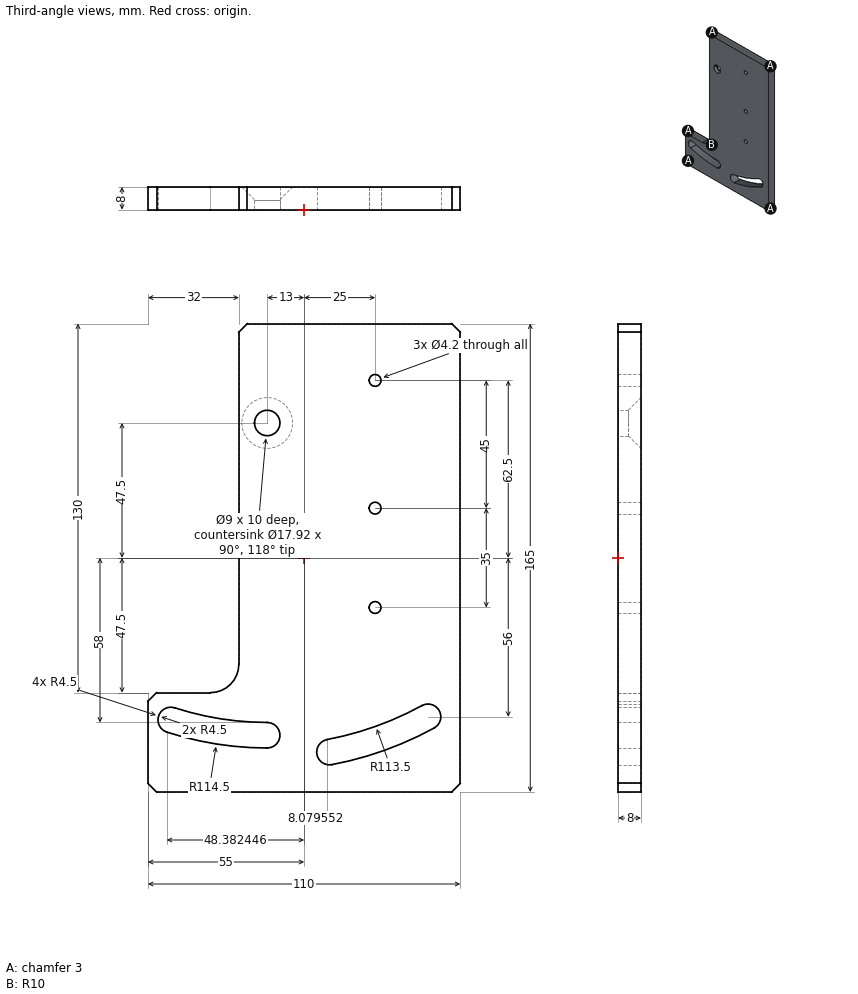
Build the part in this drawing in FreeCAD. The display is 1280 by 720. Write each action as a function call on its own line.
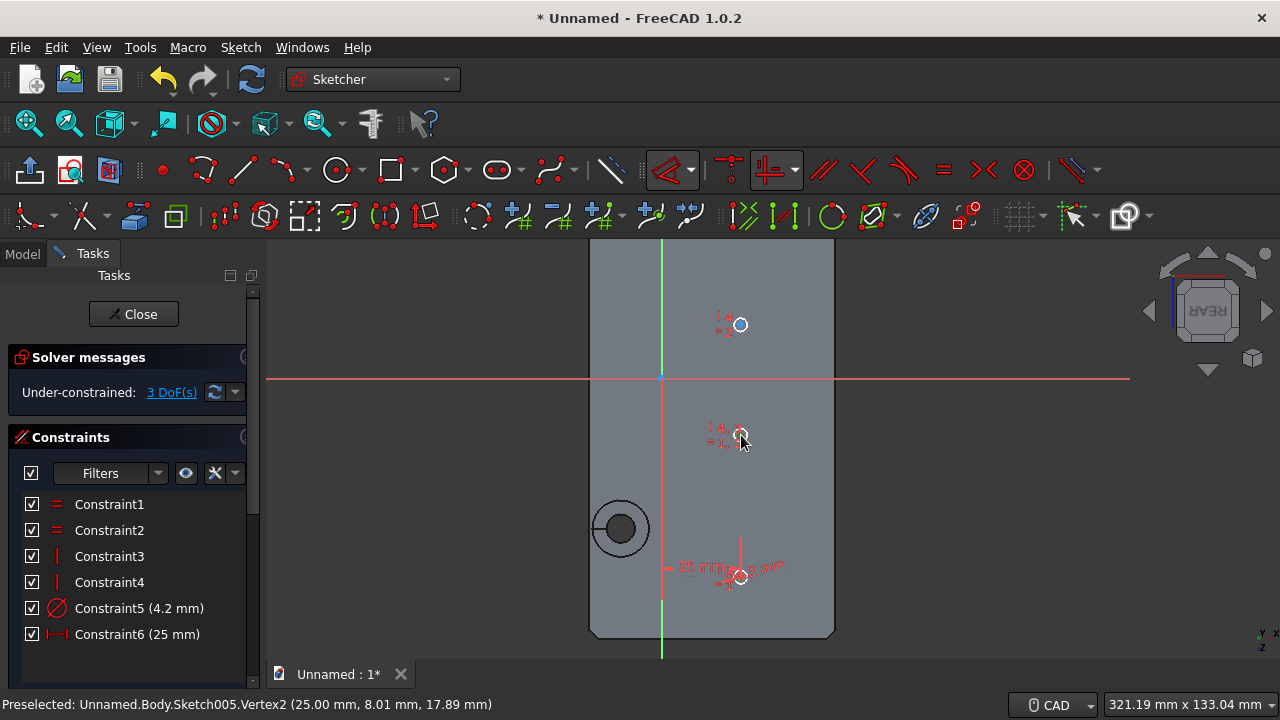
click(694, 170)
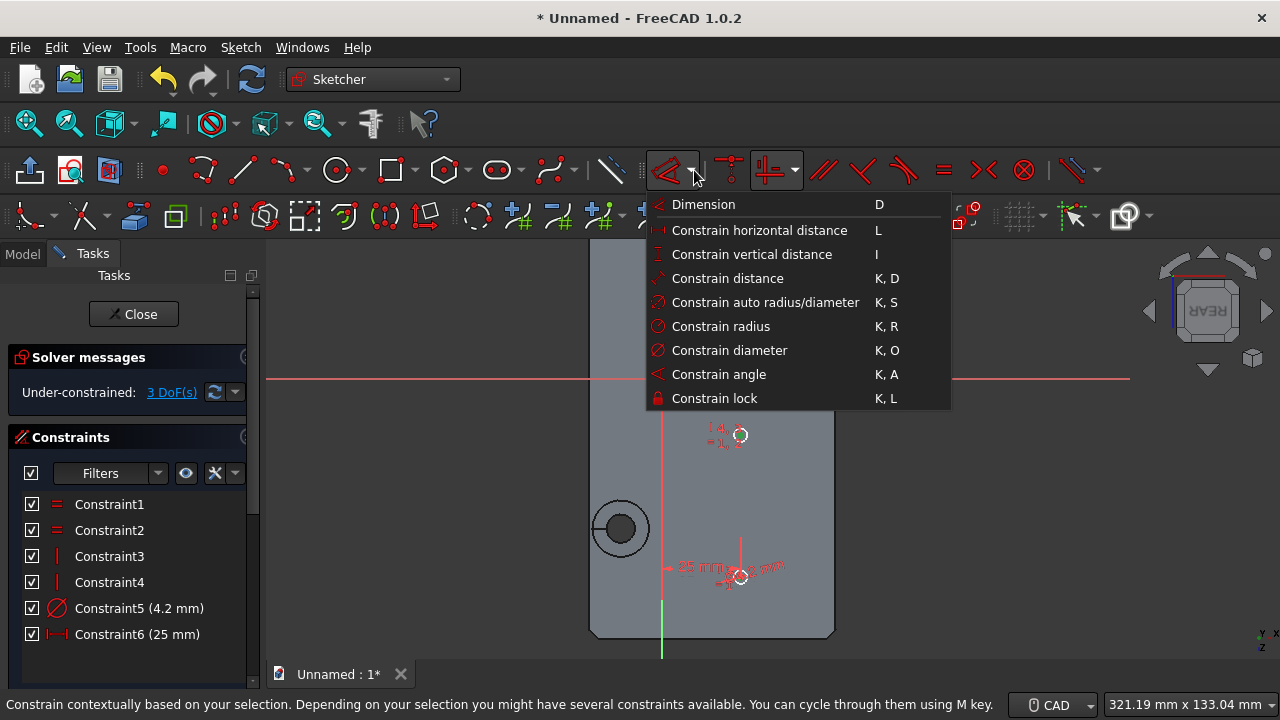
click(799, 254)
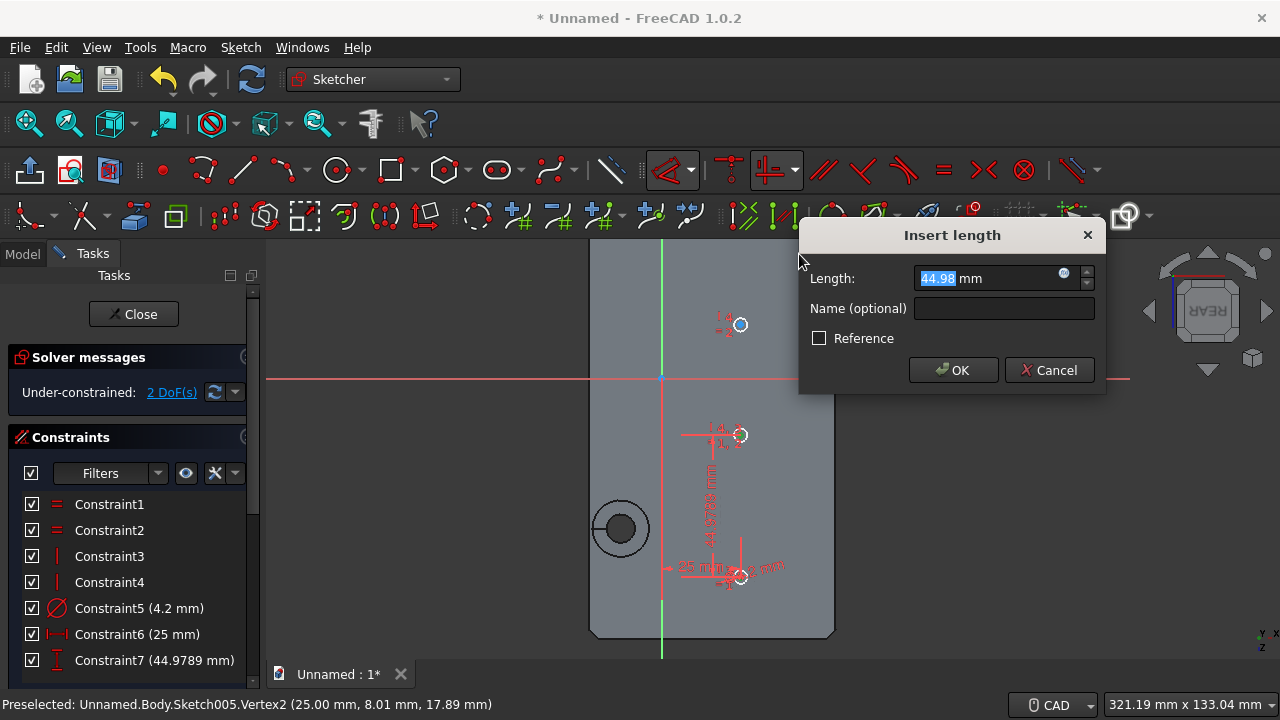
text(45)
key(Return)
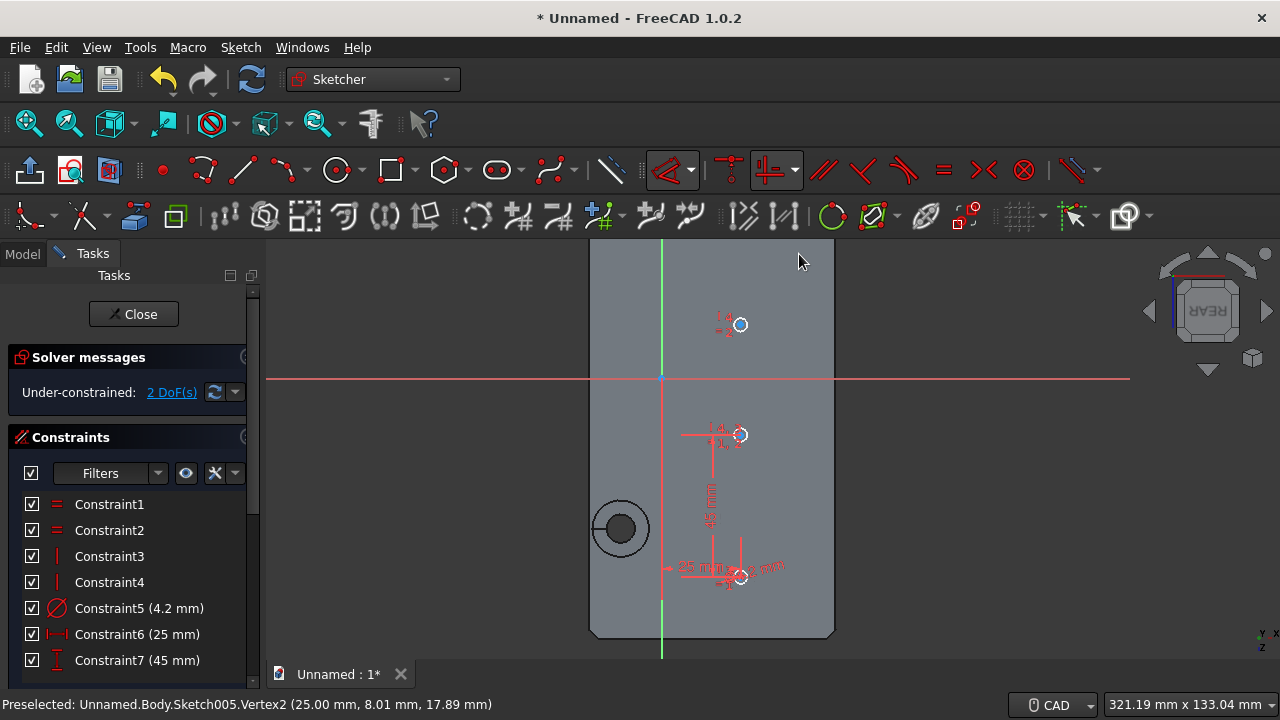
click(741, 435)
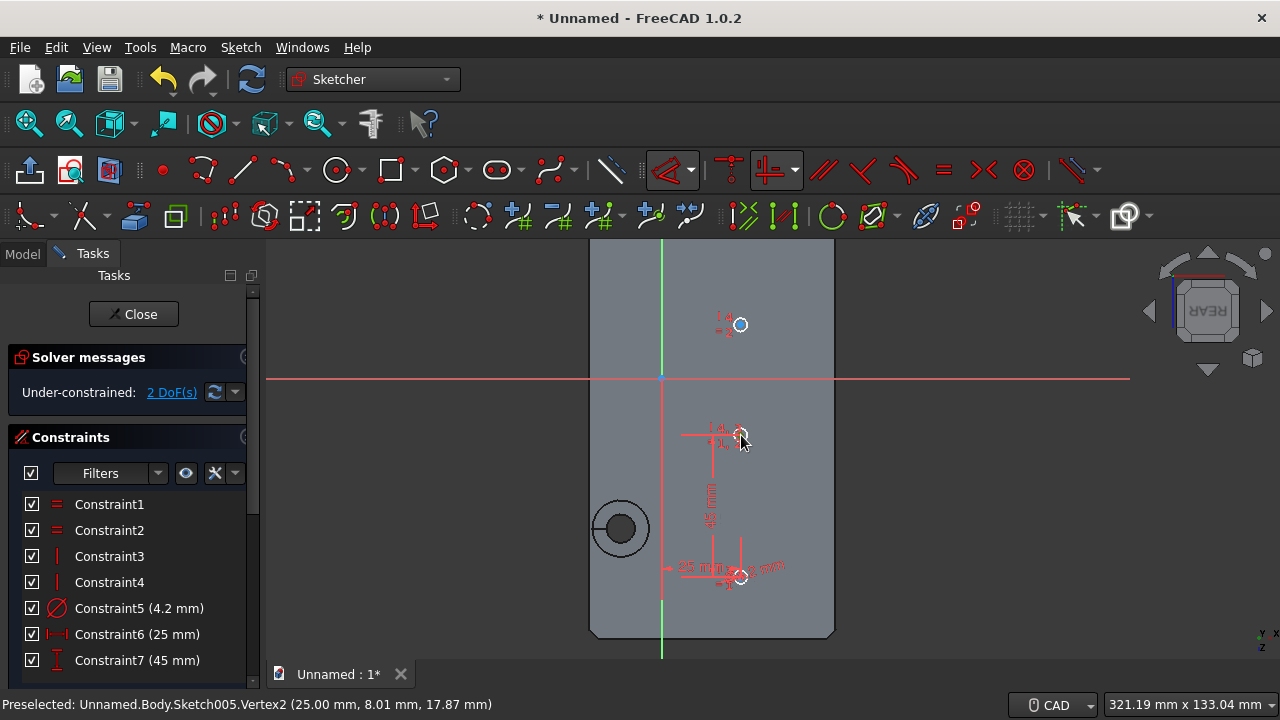
click(741, 325)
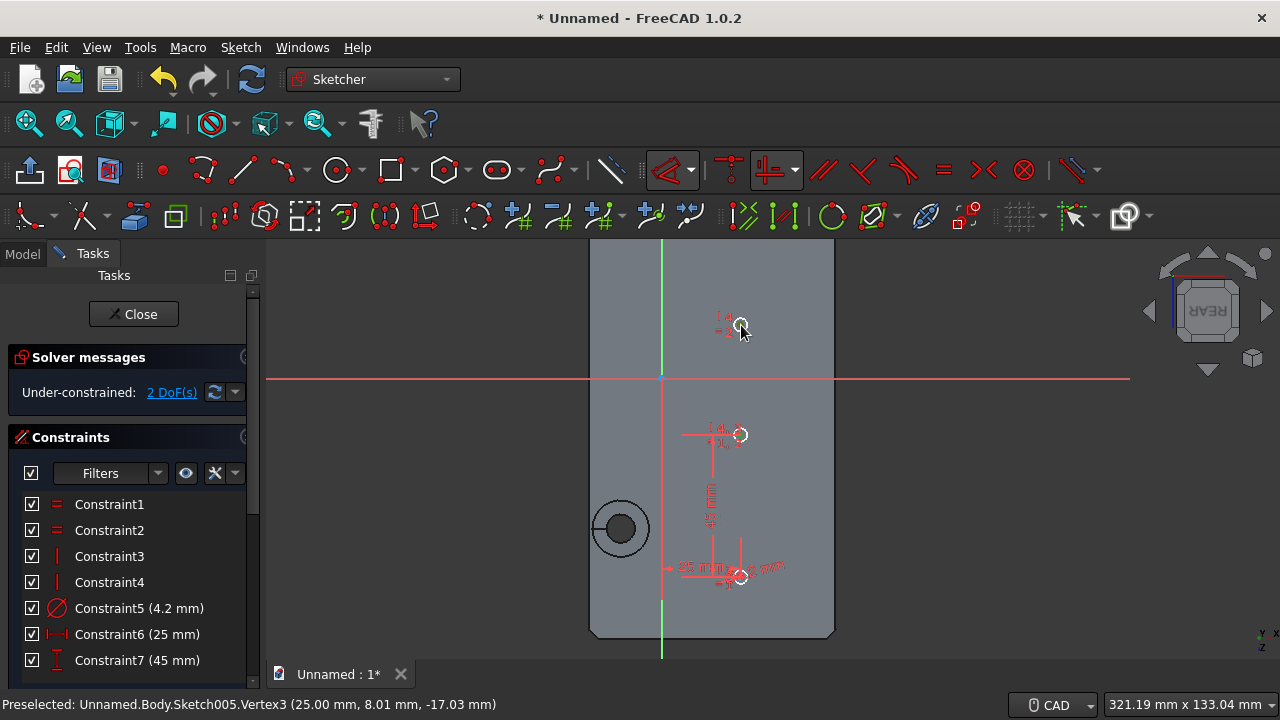
click(694, 170)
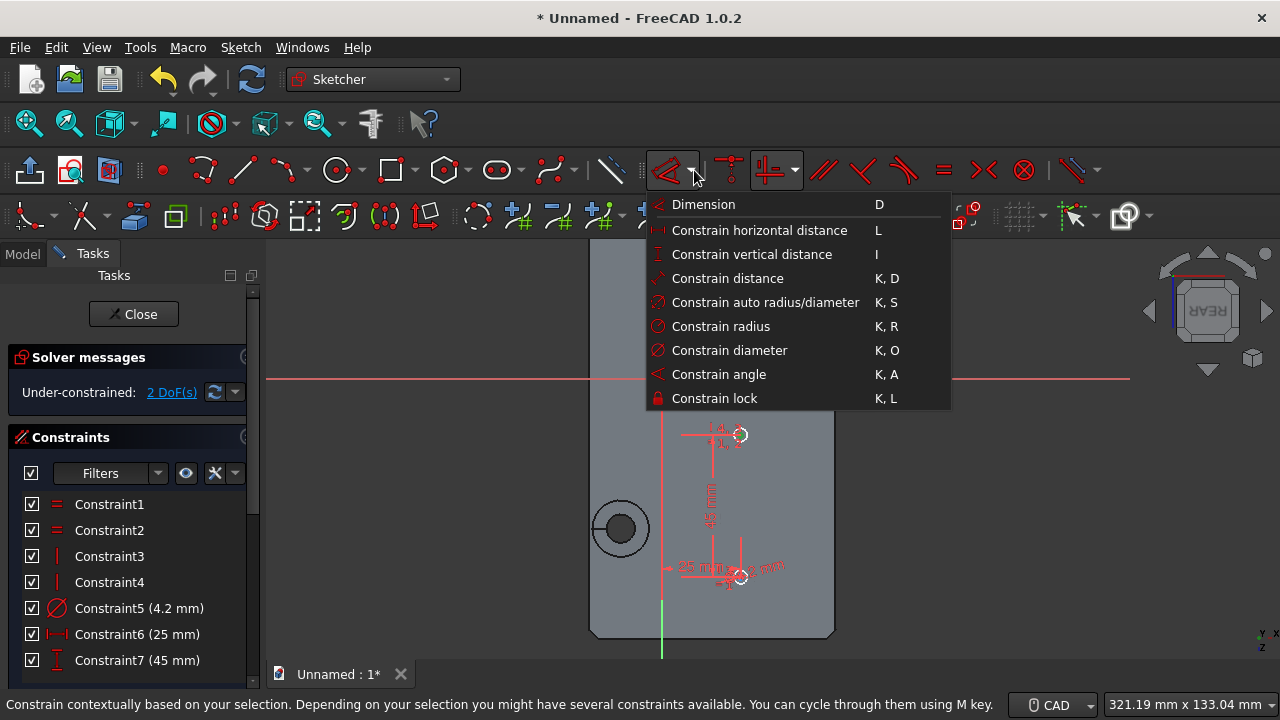
click(799, 254)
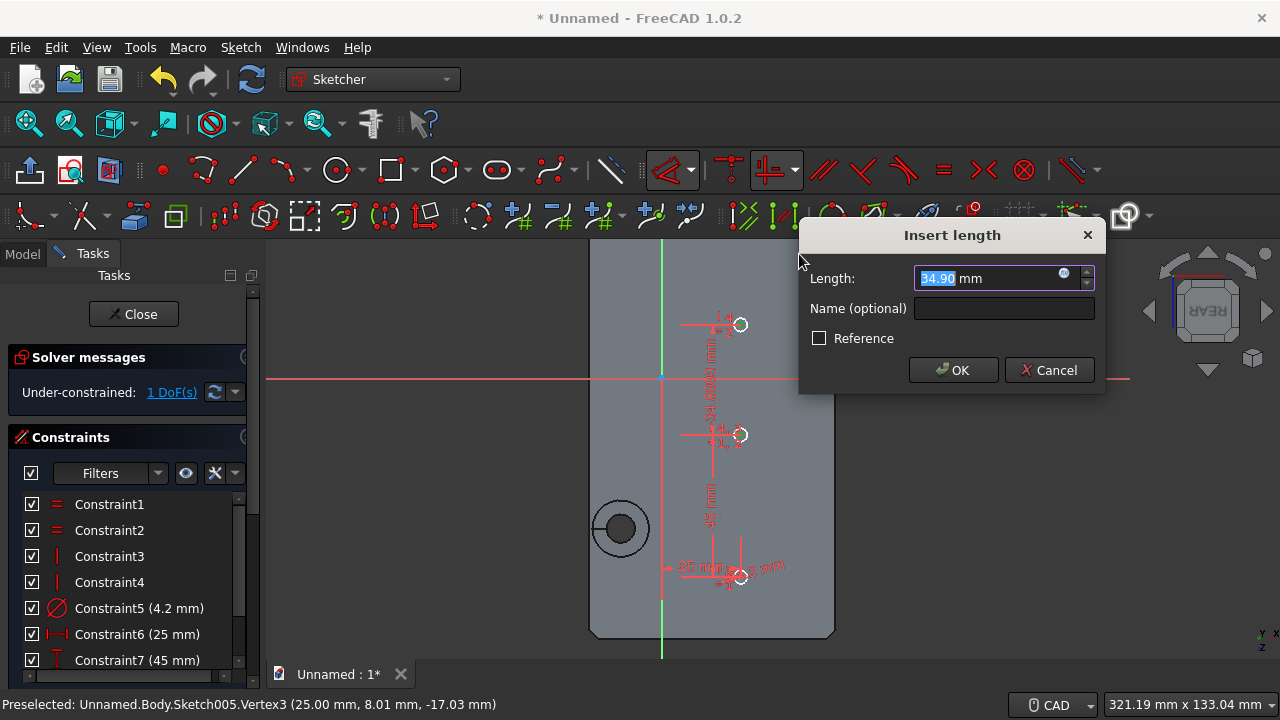
text(35)
key(Return)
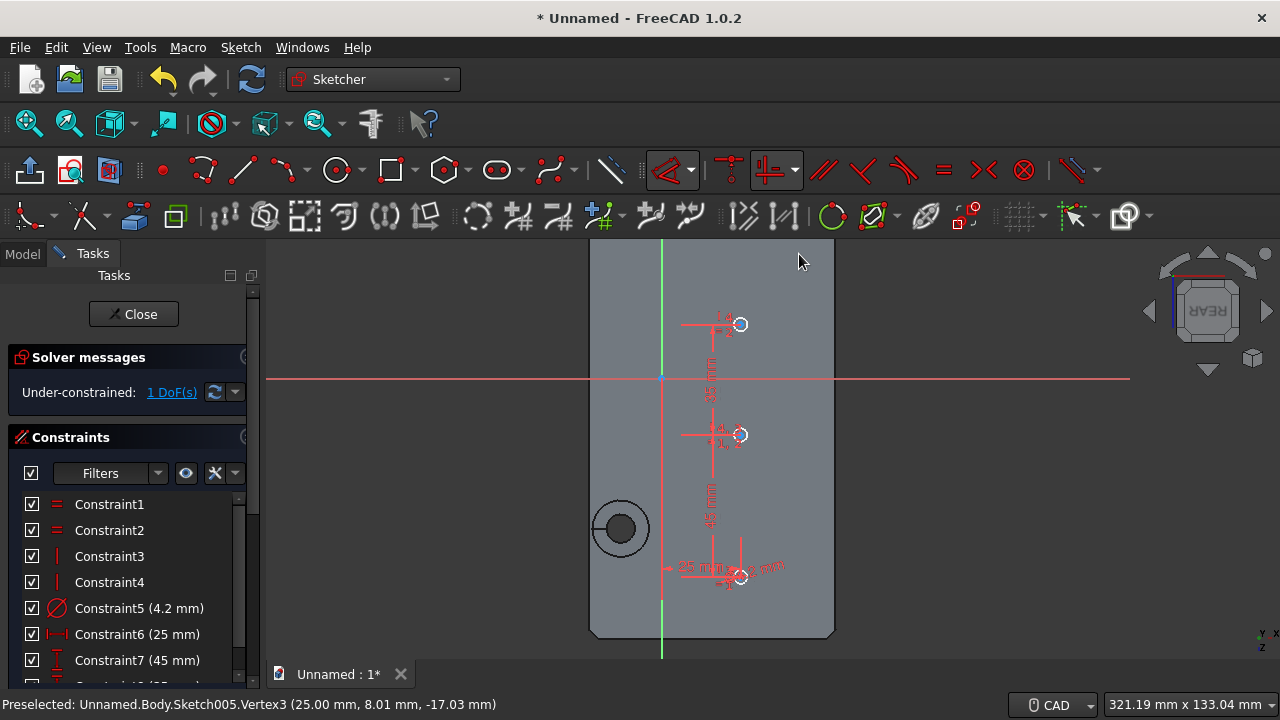
click(741, 577)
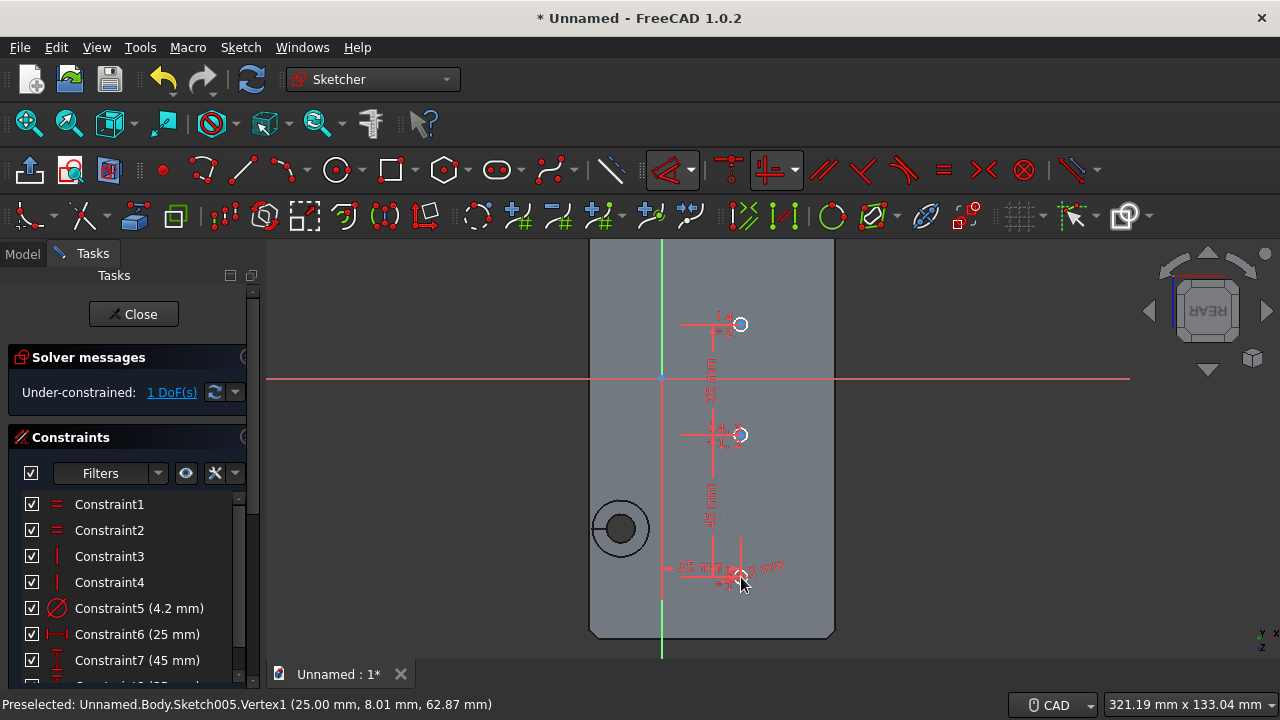
key(i)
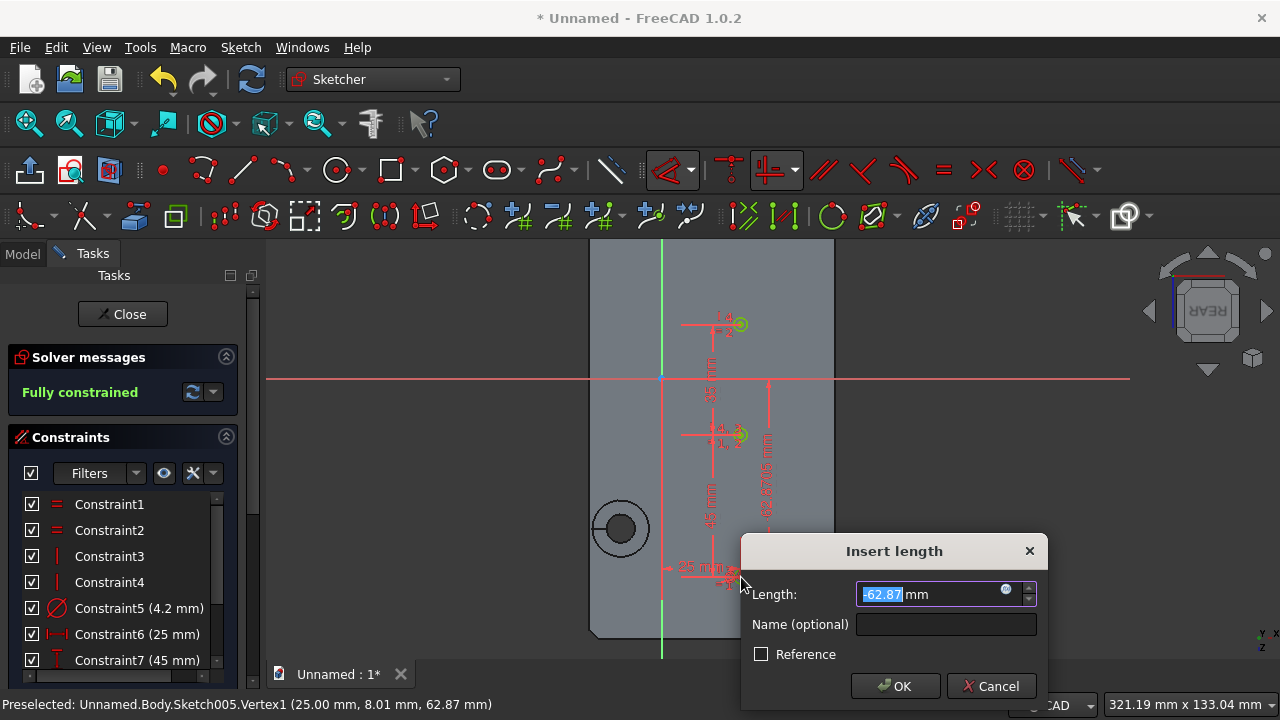
text(-62.5)
key(Return)